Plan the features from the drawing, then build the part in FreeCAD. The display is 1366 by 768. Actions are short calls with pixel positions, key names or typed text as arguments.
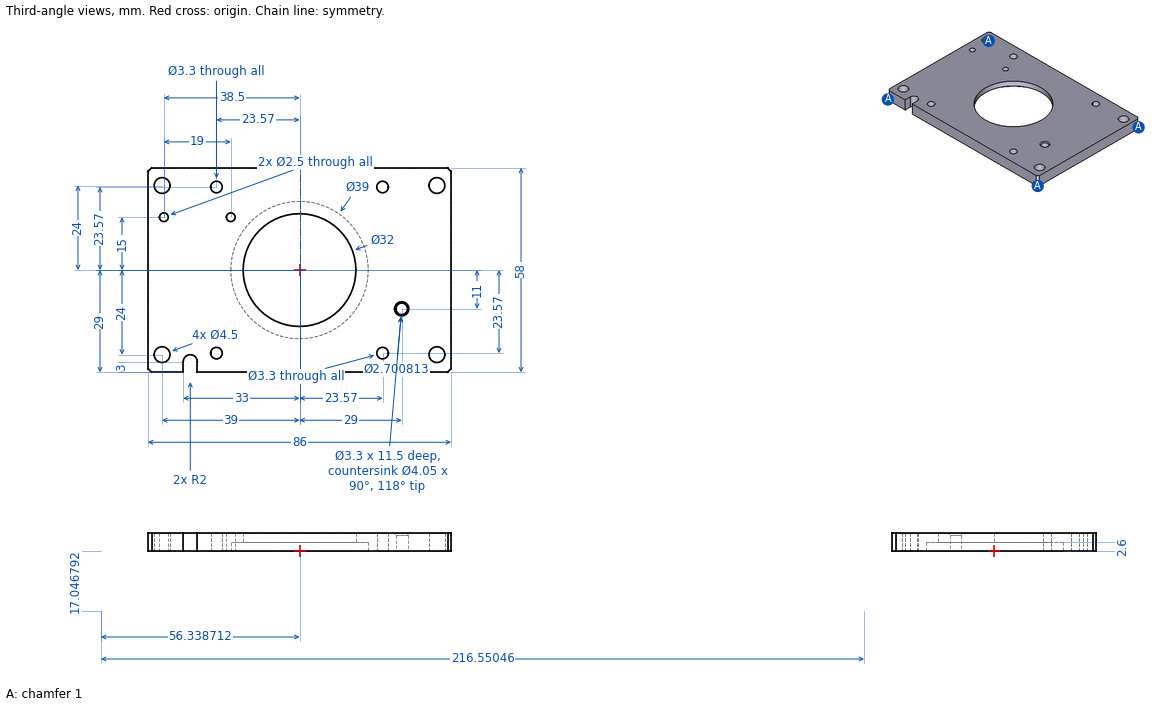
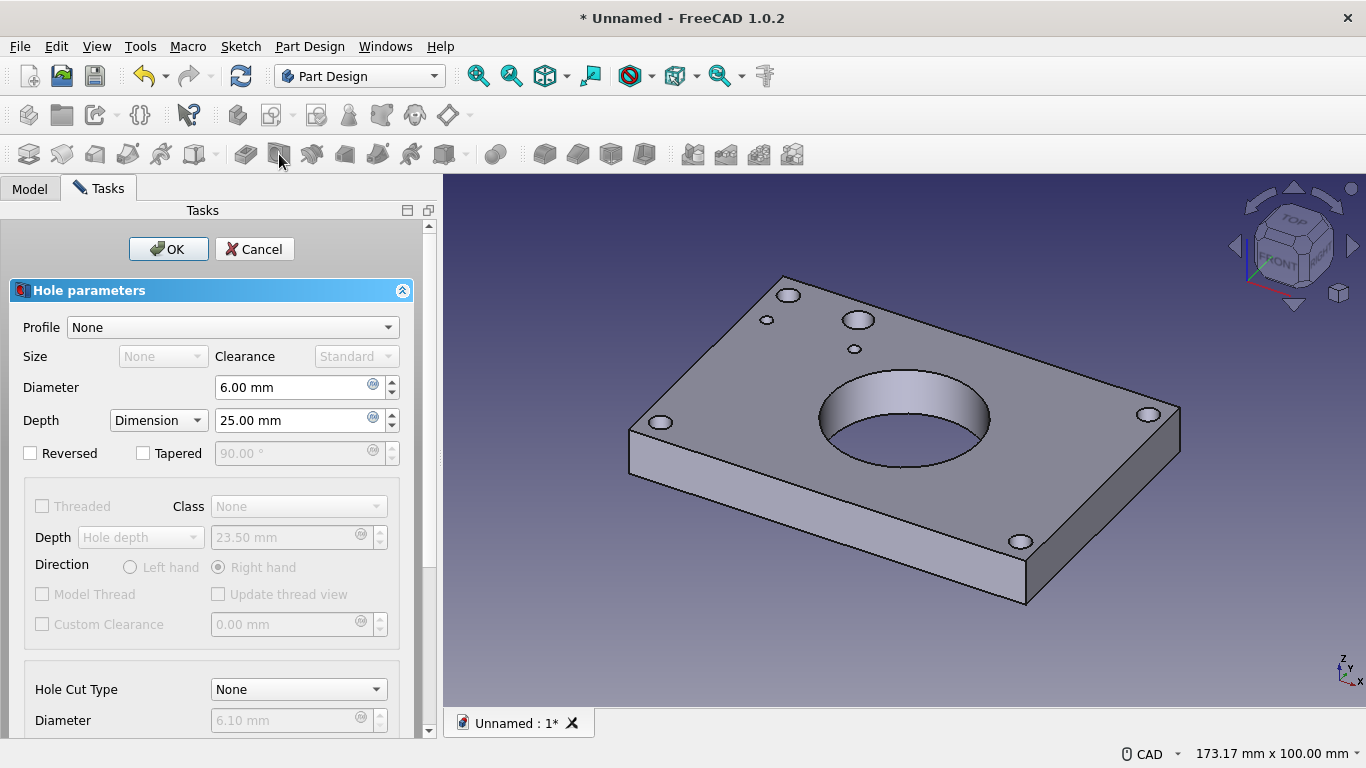
triple_click(300, 388)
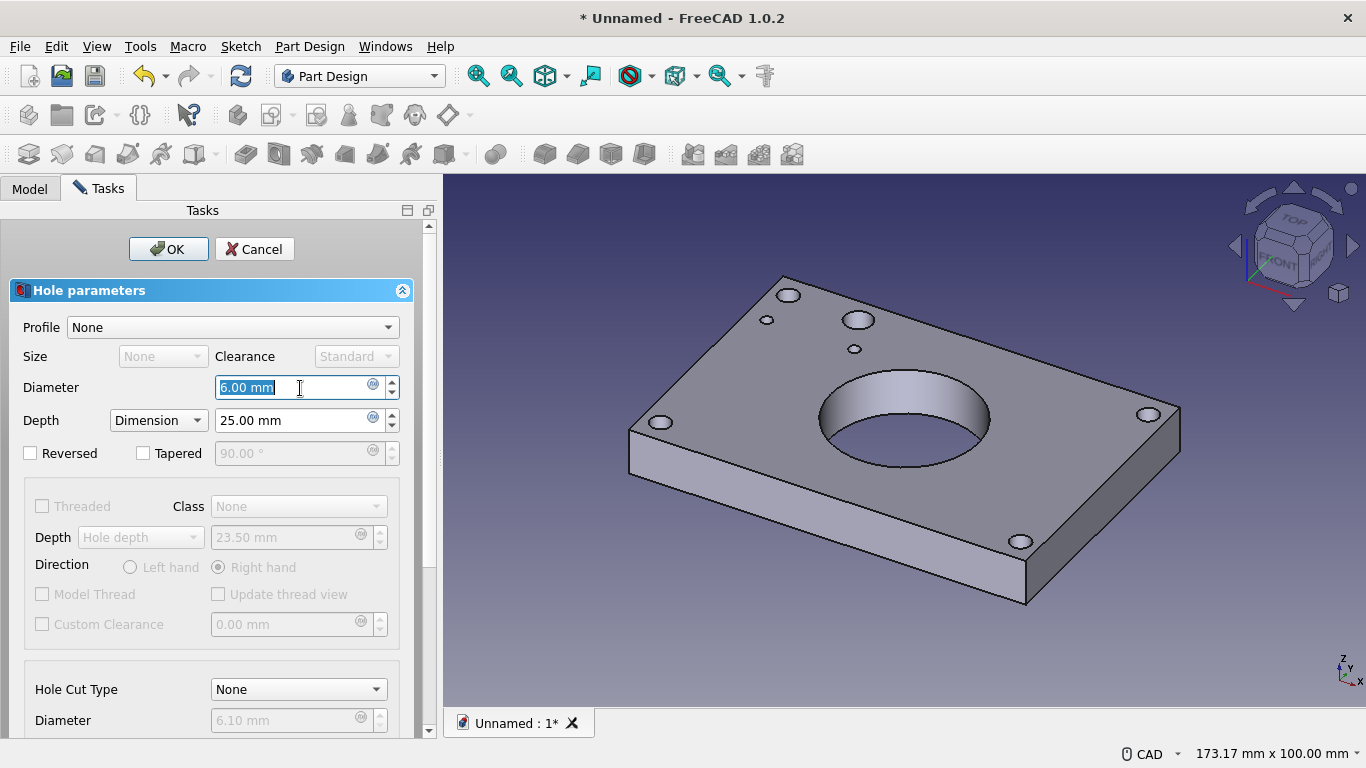
text(3.3)
key(Tab)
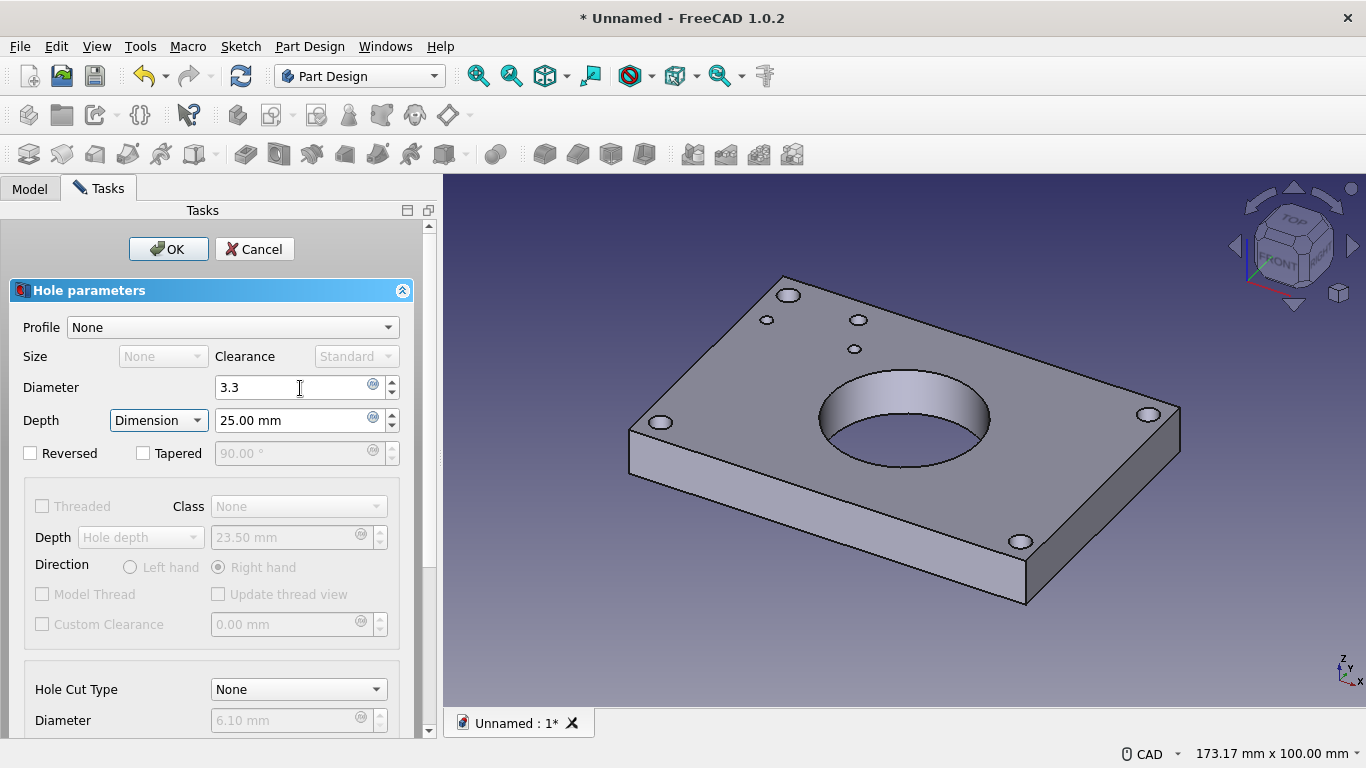
click(160, 420)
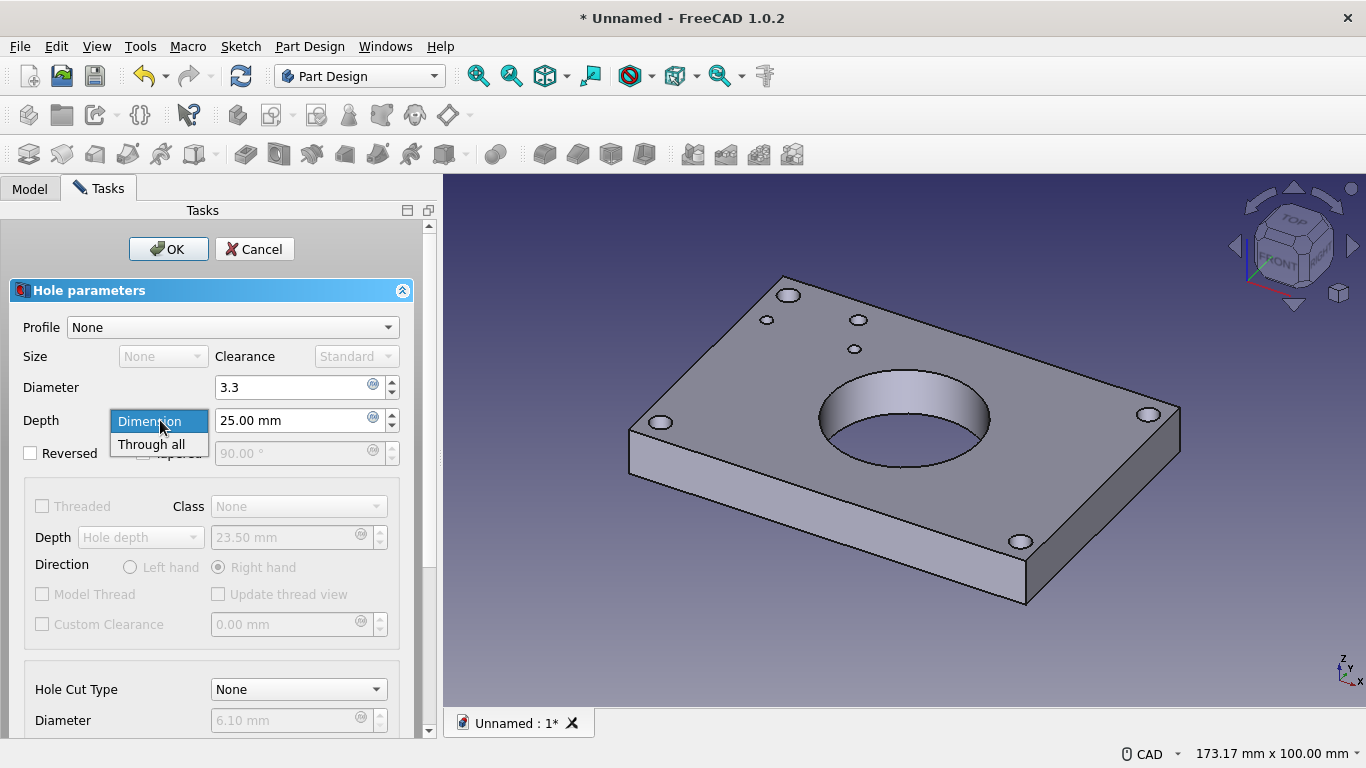
click(158, 444)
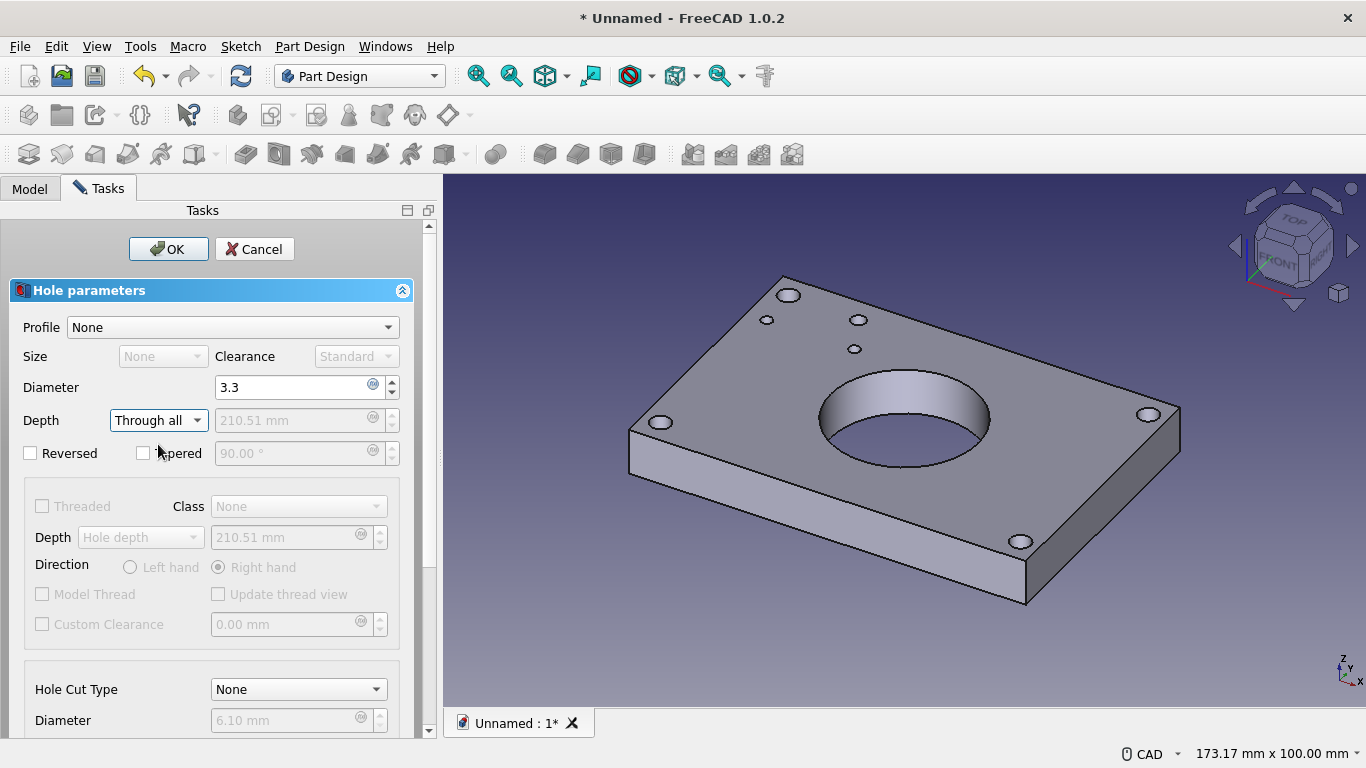
click(169, 249)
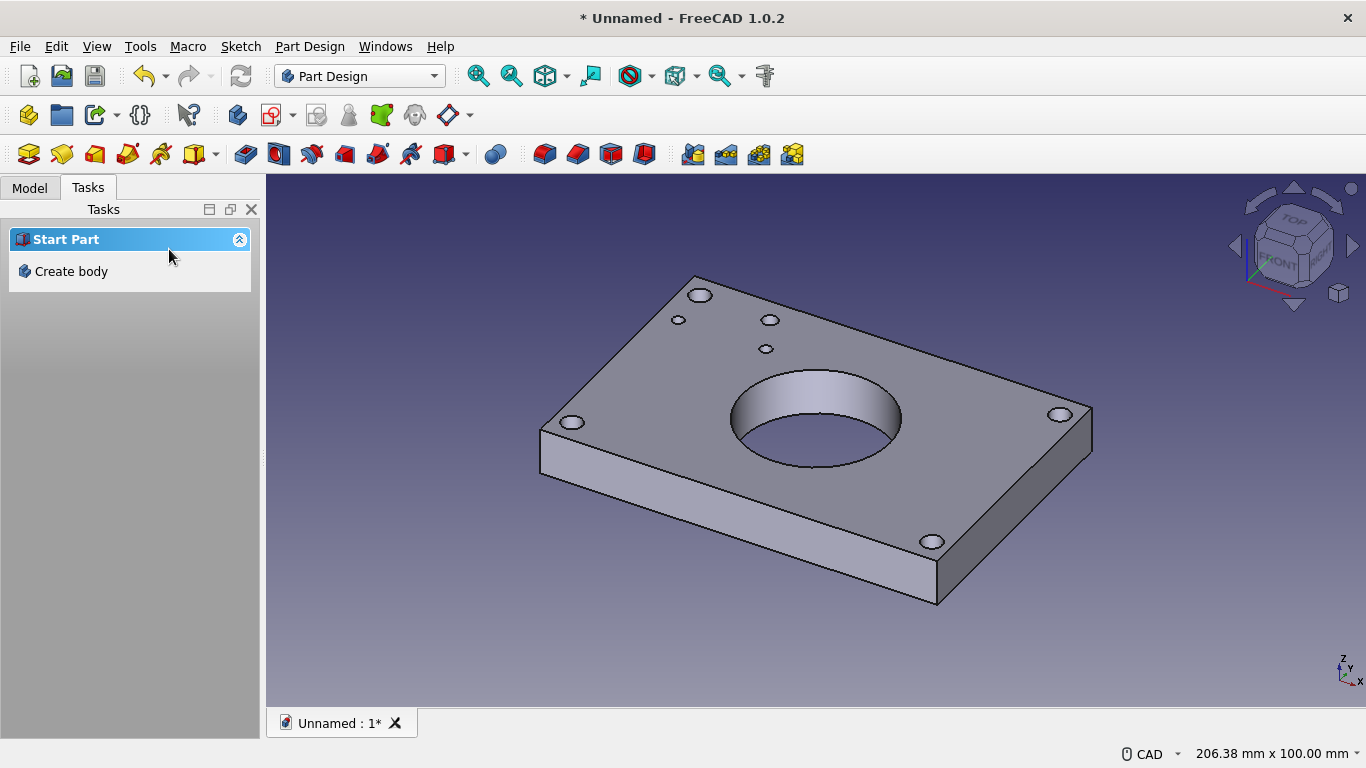
click(30, 188)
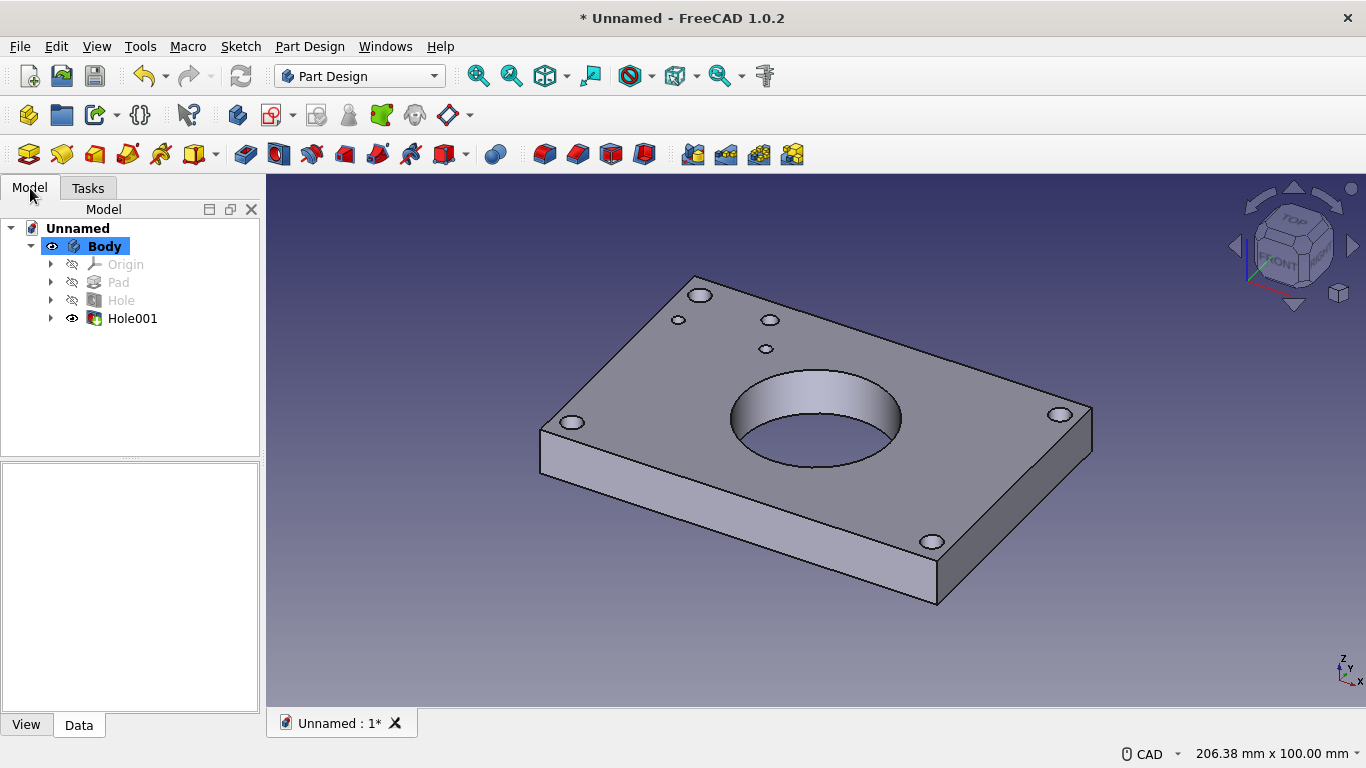
click(117, 318)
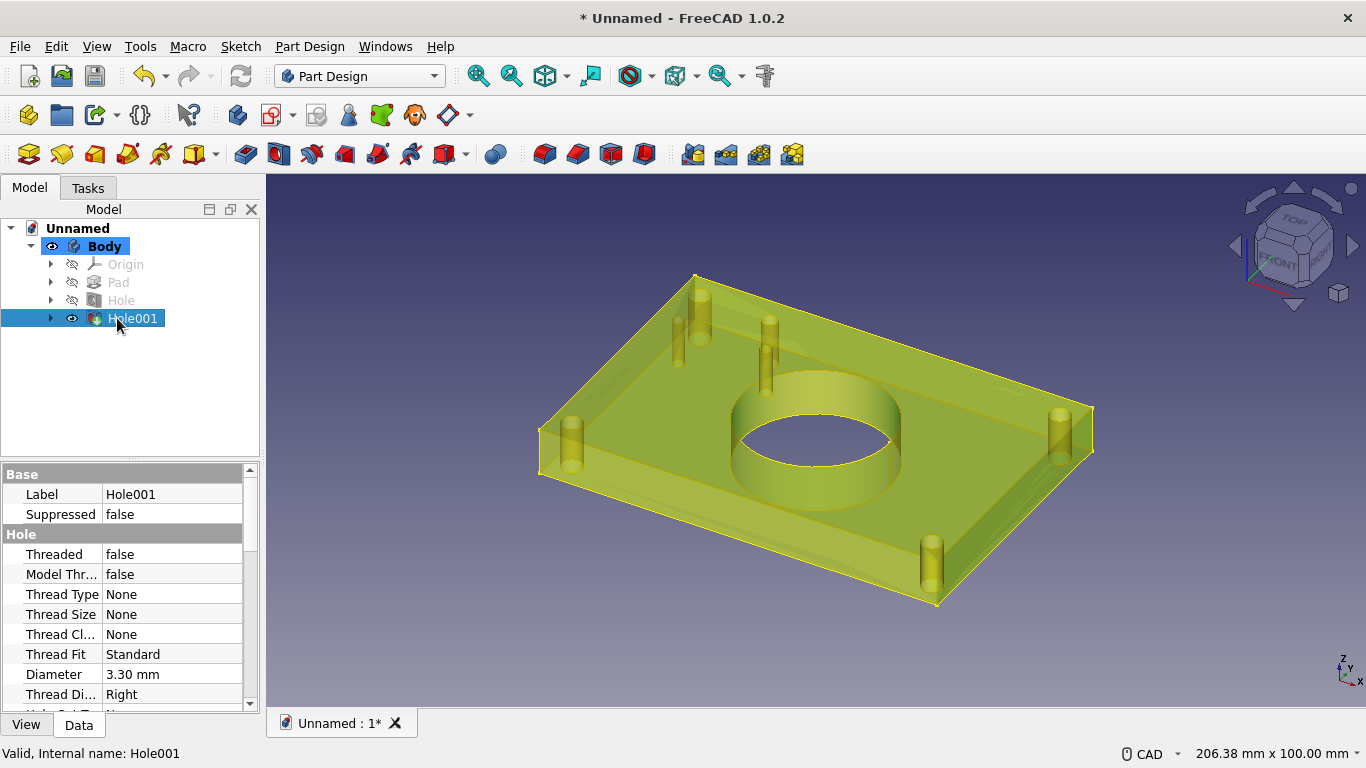
click(693, 154)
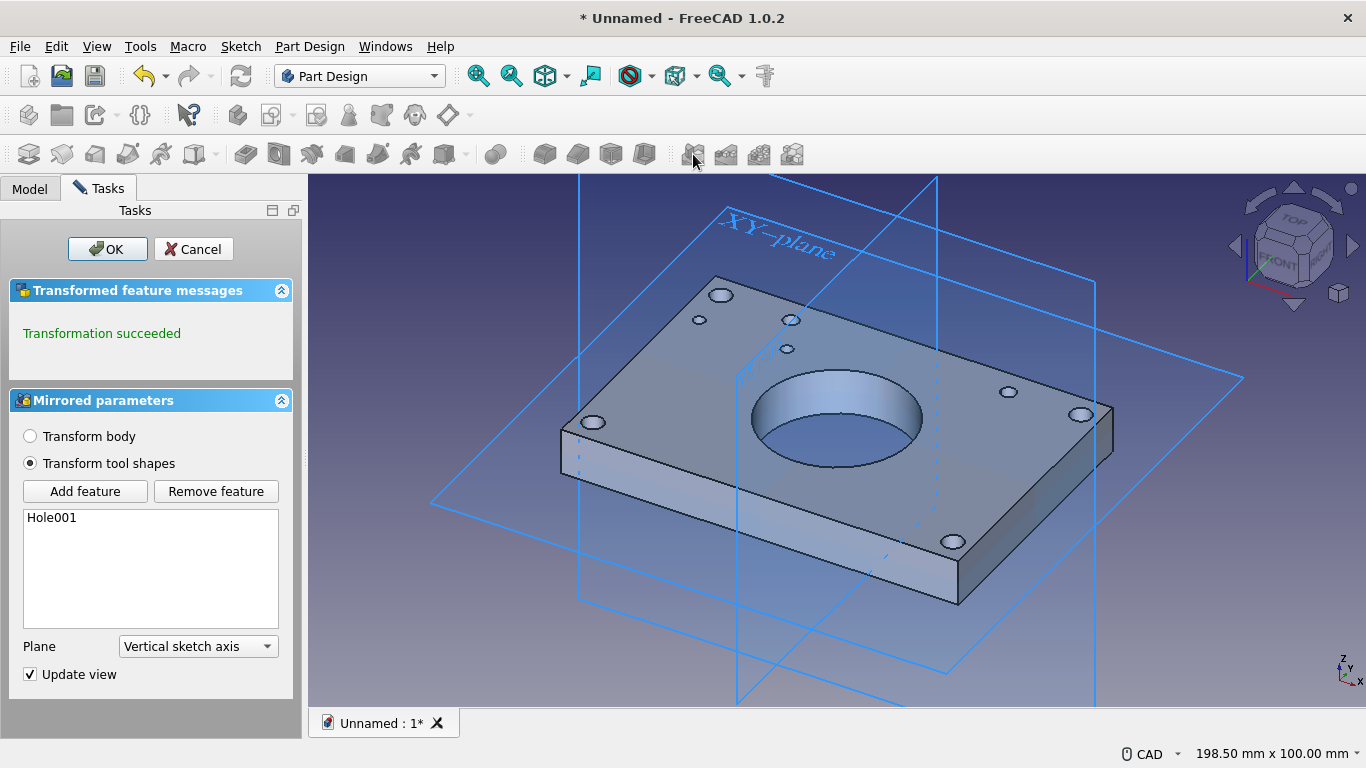
click(199, 646)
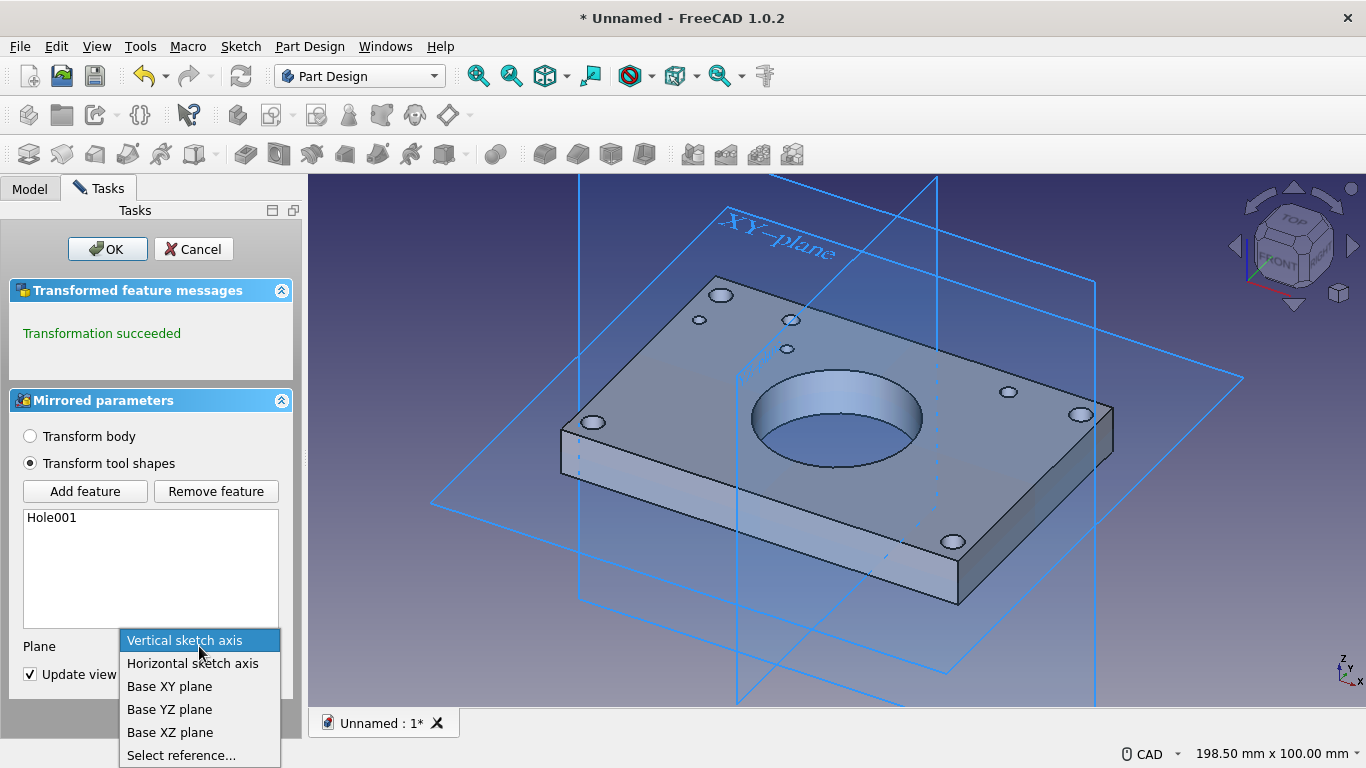
click(198, 732)